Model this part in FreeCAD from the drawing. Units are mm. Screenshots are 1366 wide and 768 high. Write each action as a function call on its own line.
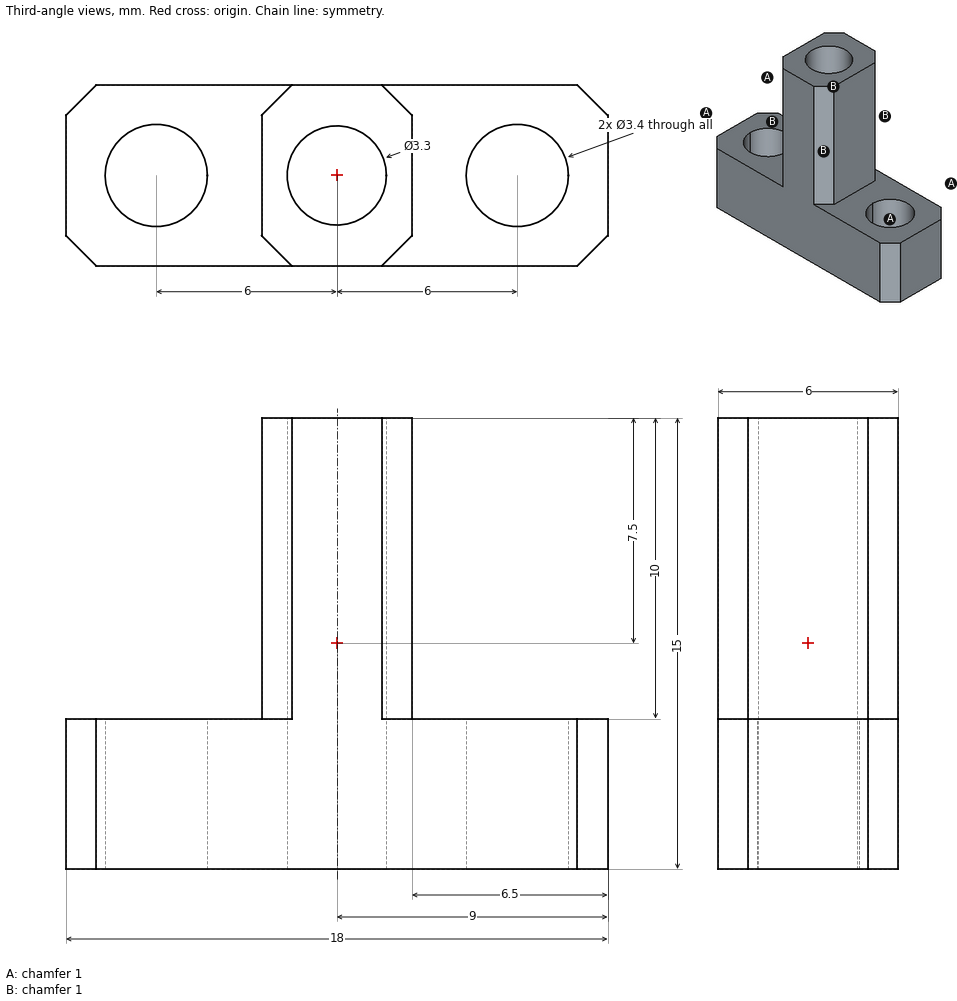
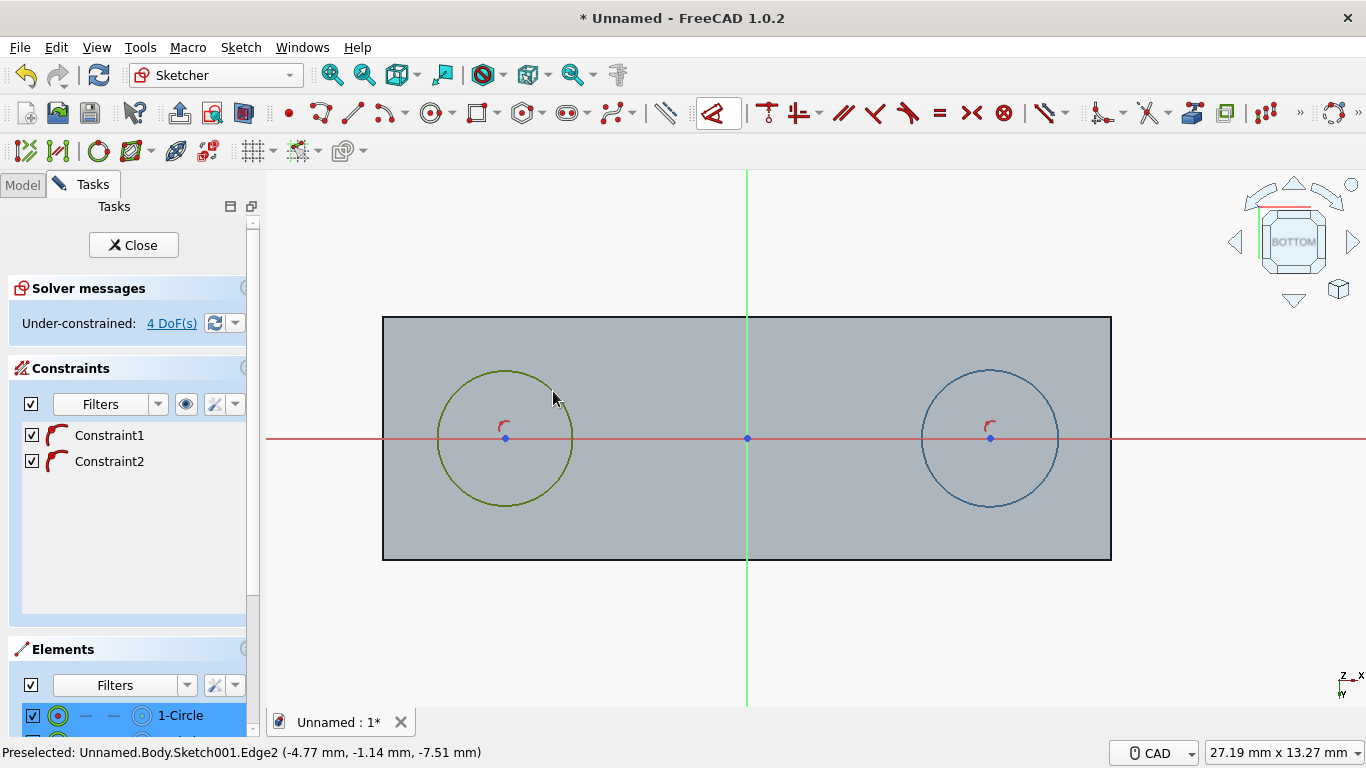
click(940, 114)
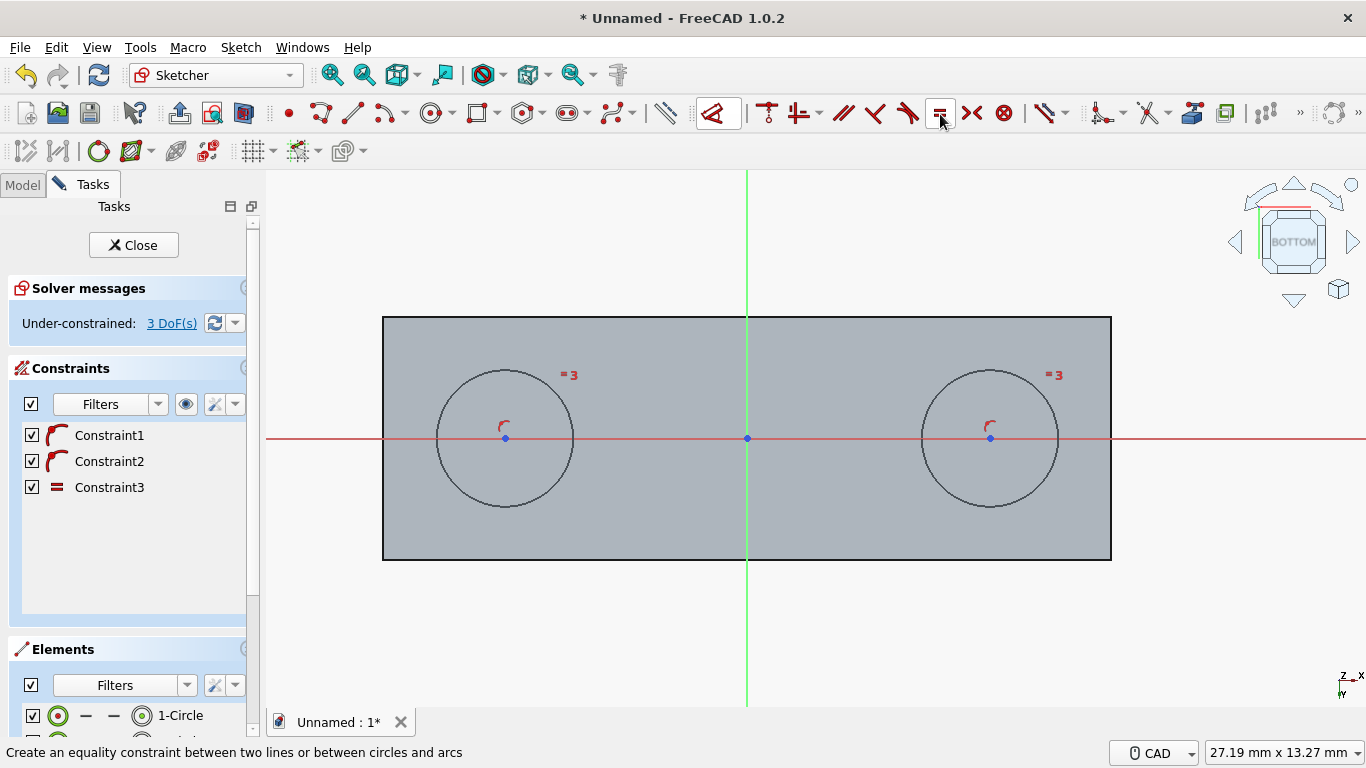
click(1038, 390)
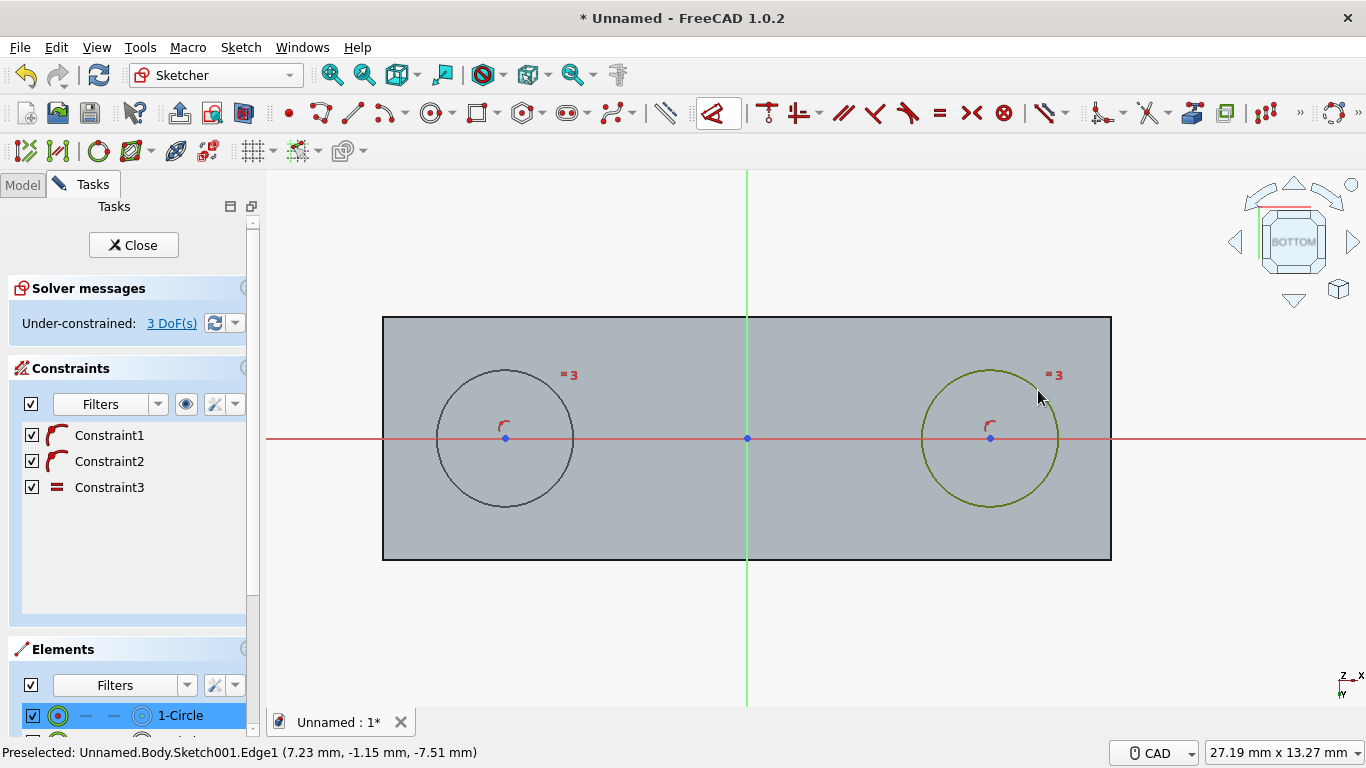
click(736, 114)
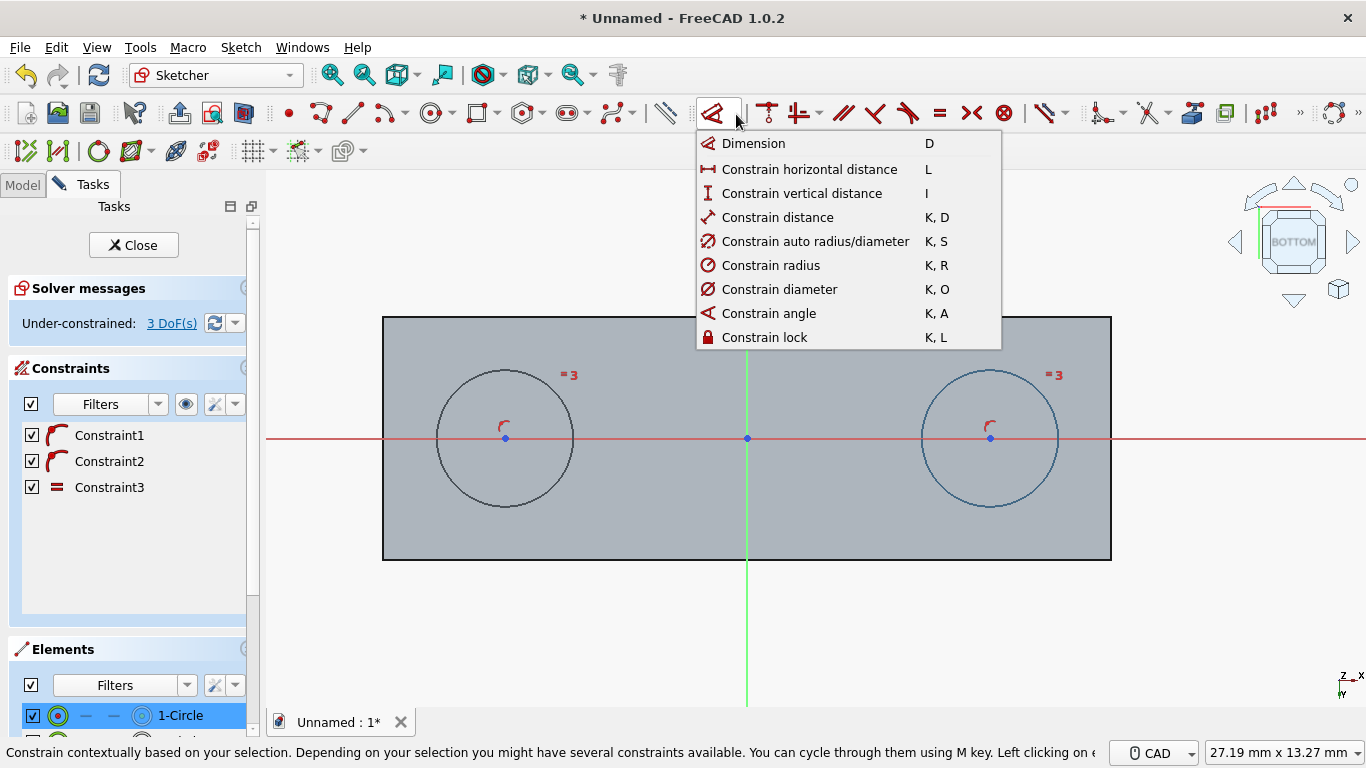
click(849, 289)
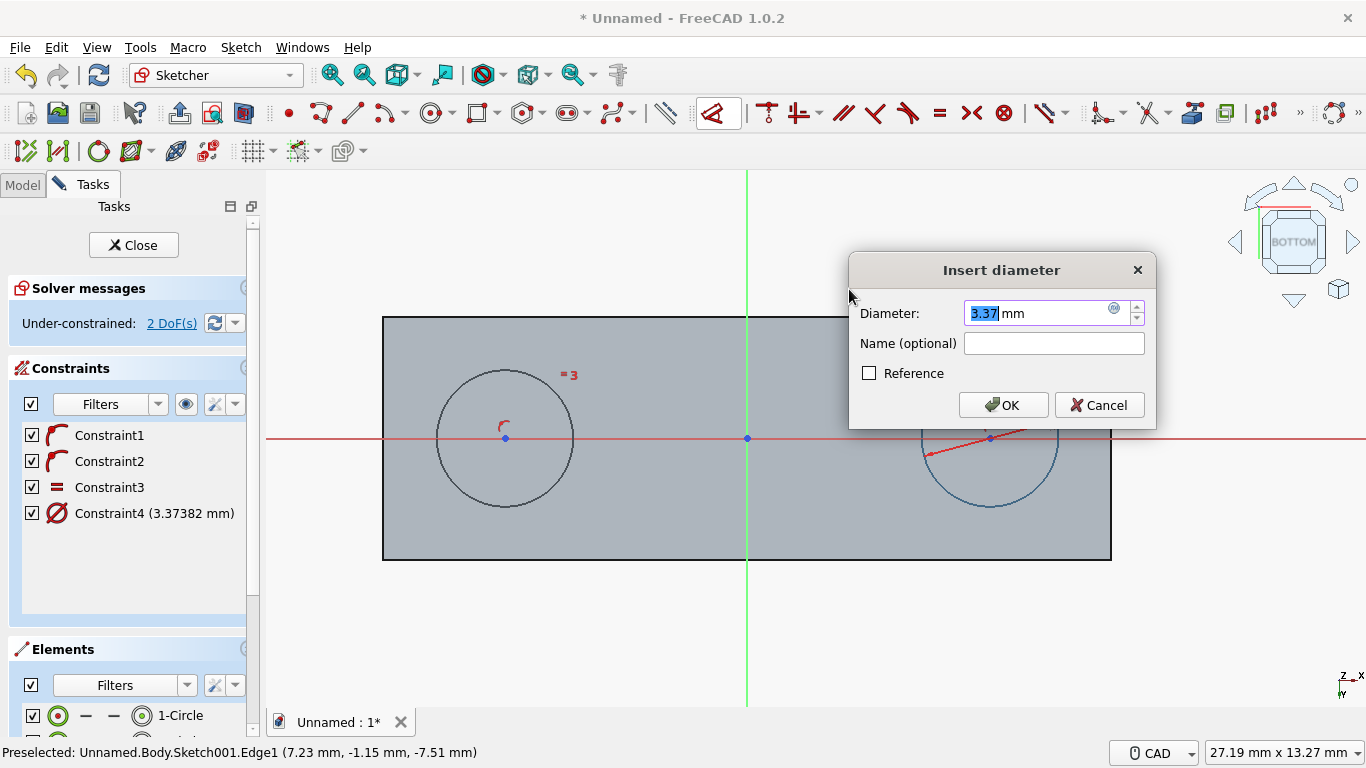
text(3.4)
key(Return)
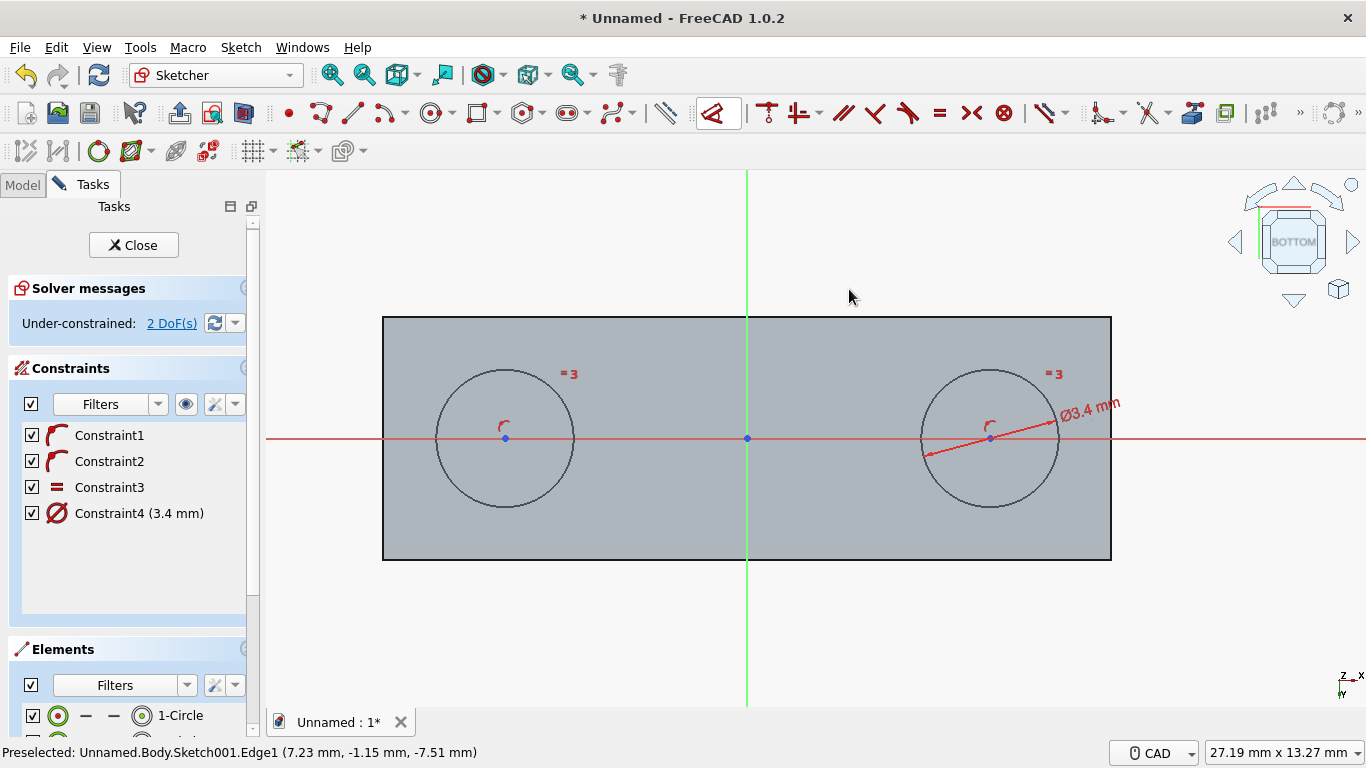
click(990, 438)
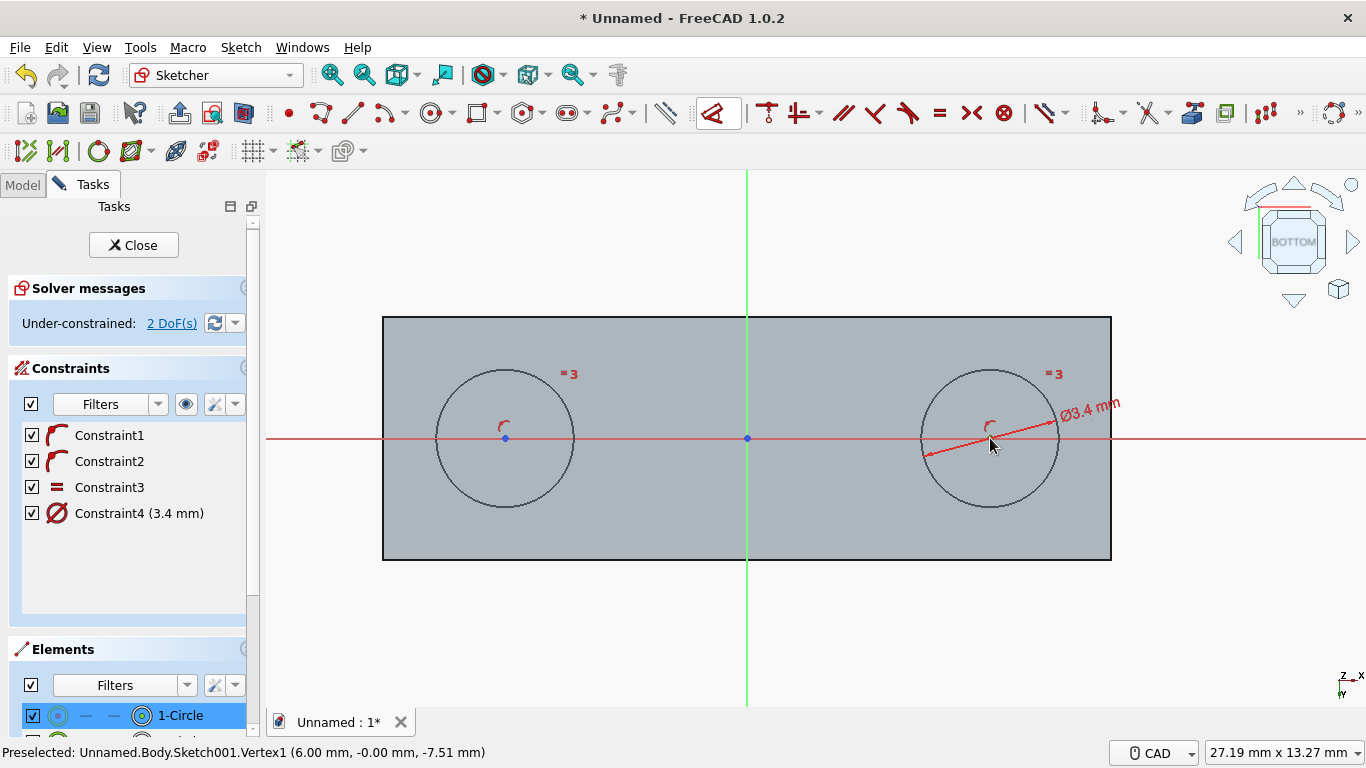
click(736, 114)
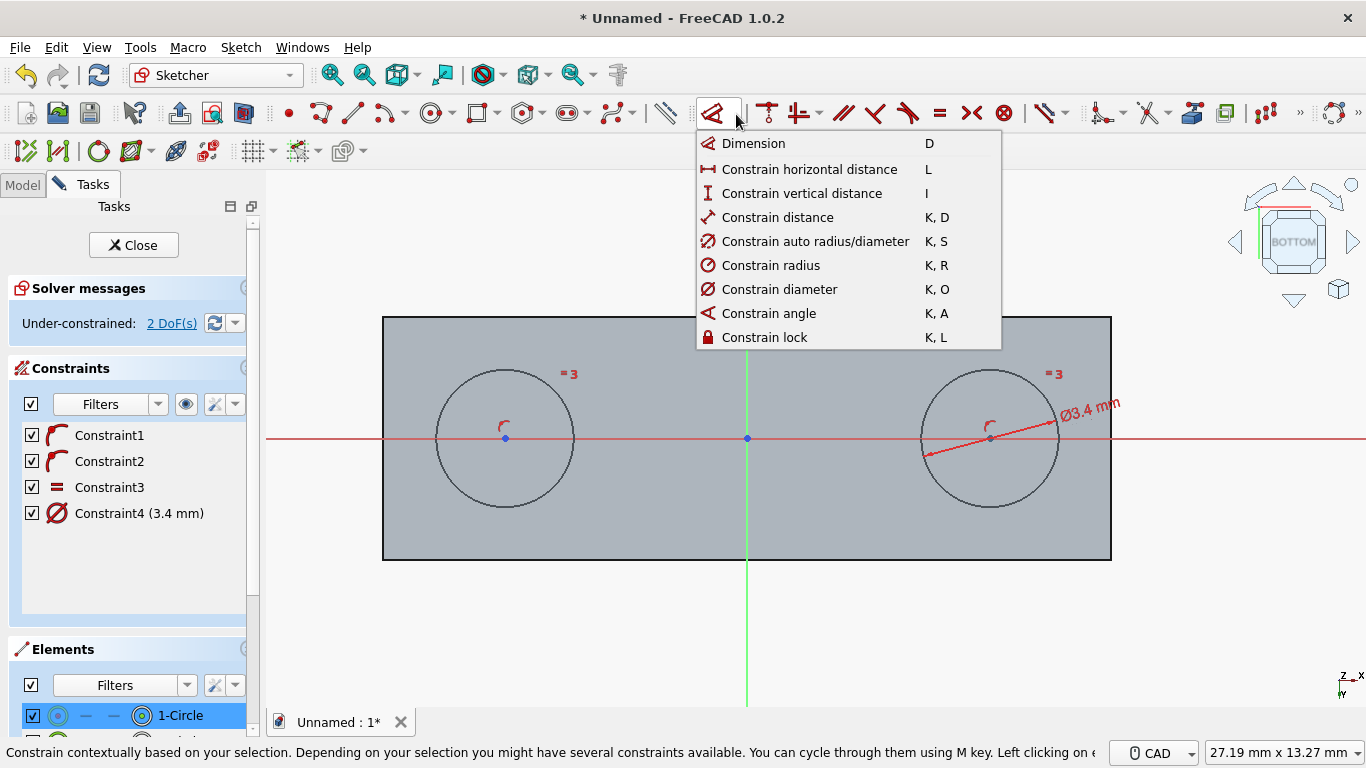
click(849, 169)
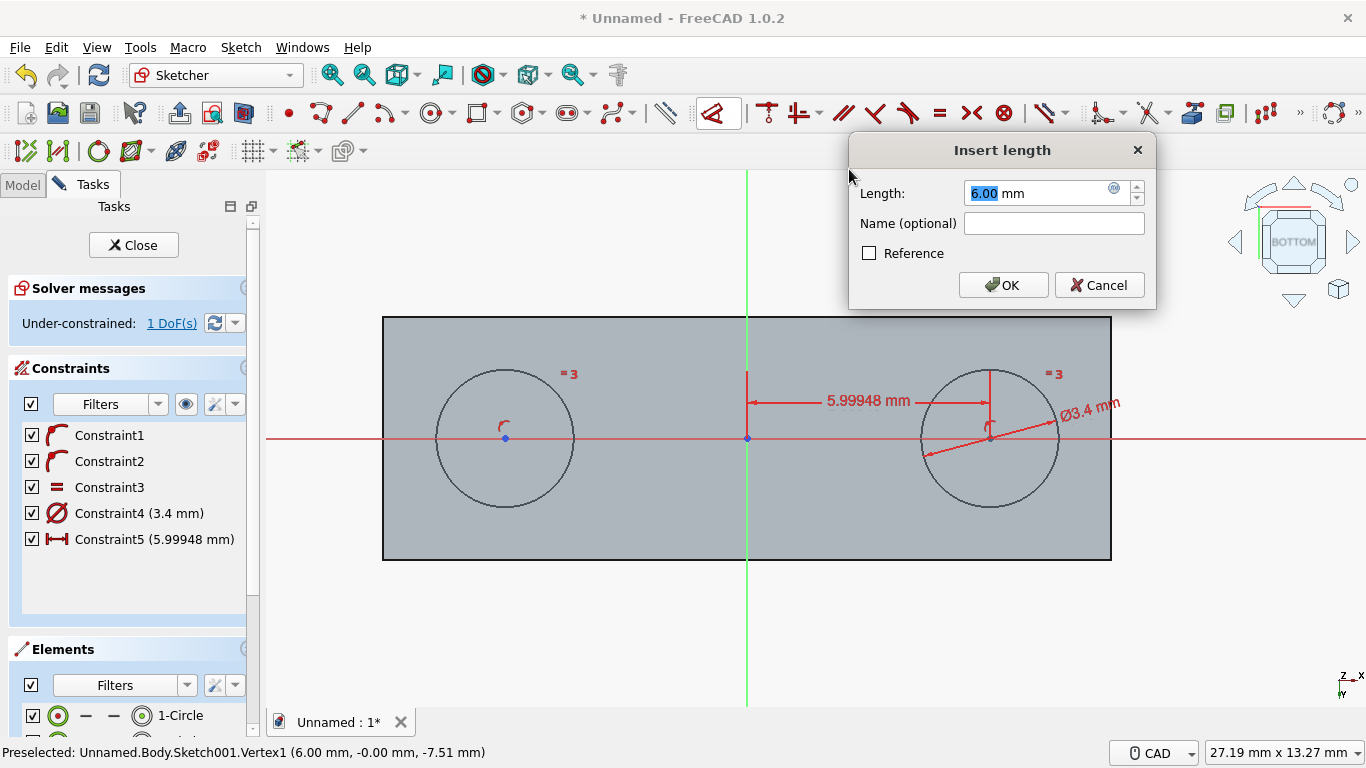
text(6)
key(Return)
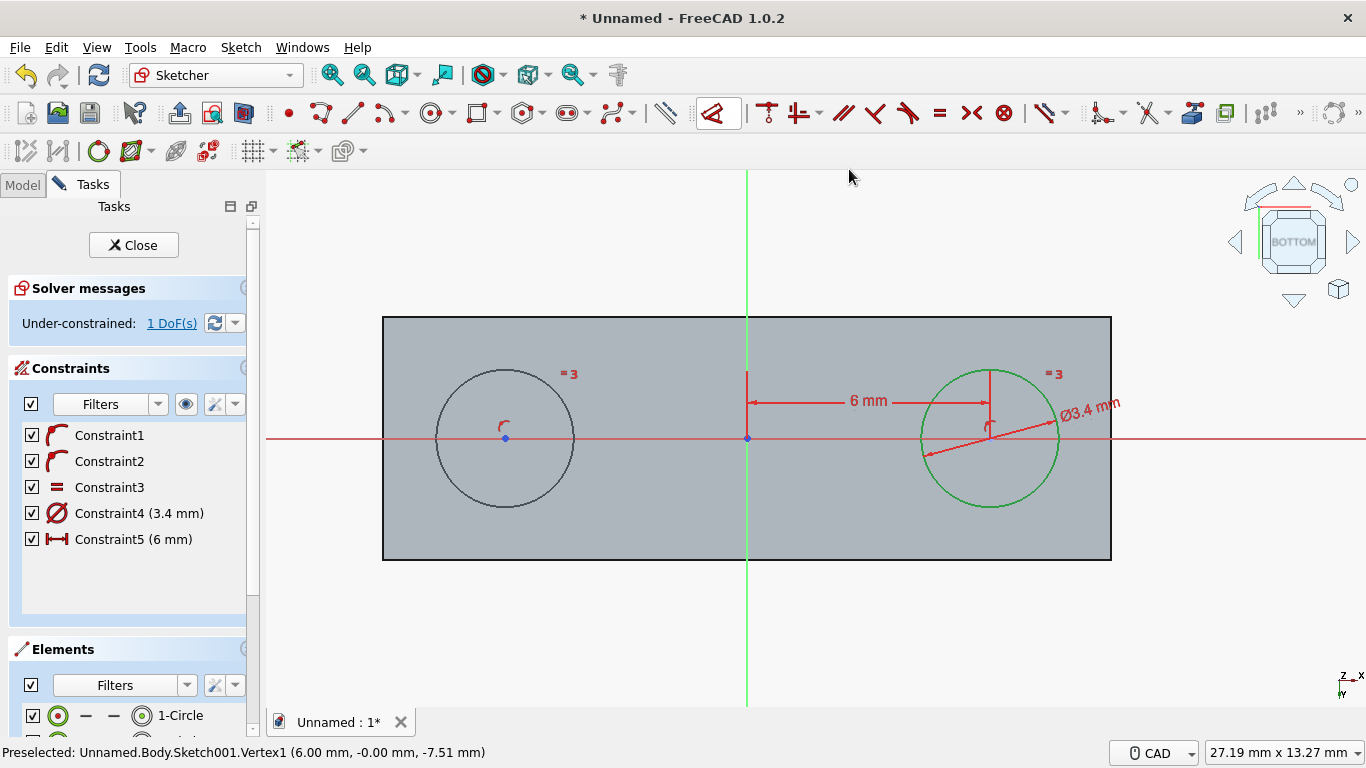
click(505, 438)